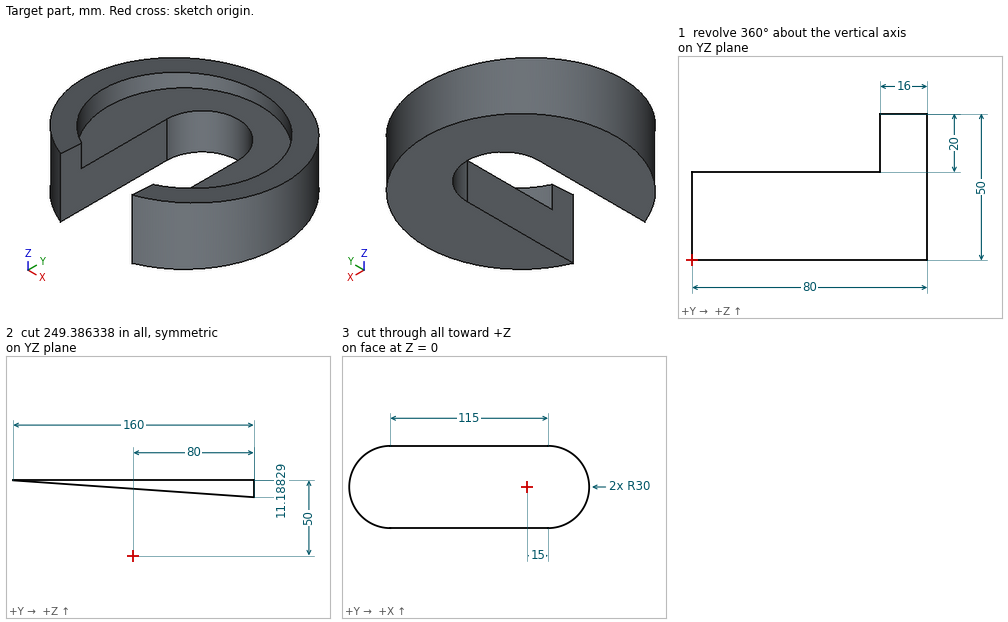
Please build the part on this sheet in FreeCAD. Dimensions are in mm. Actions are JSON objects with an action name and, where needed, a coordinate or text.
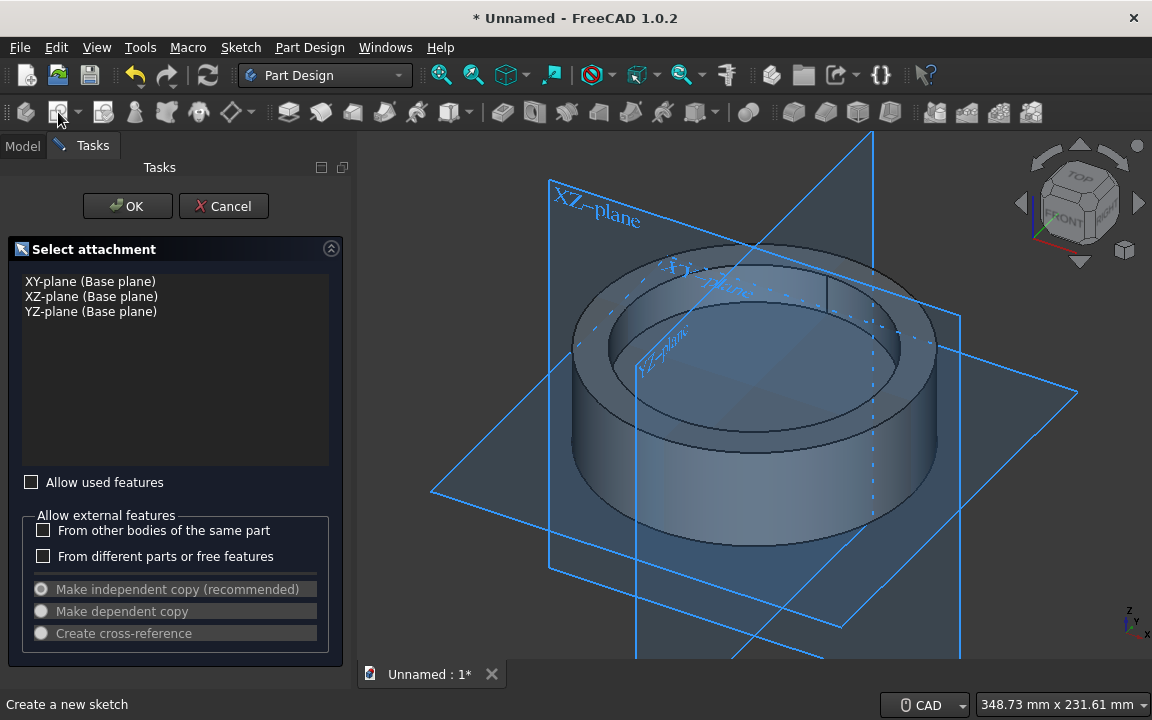
{"action": "left_click", "coordinate": [82, 312]}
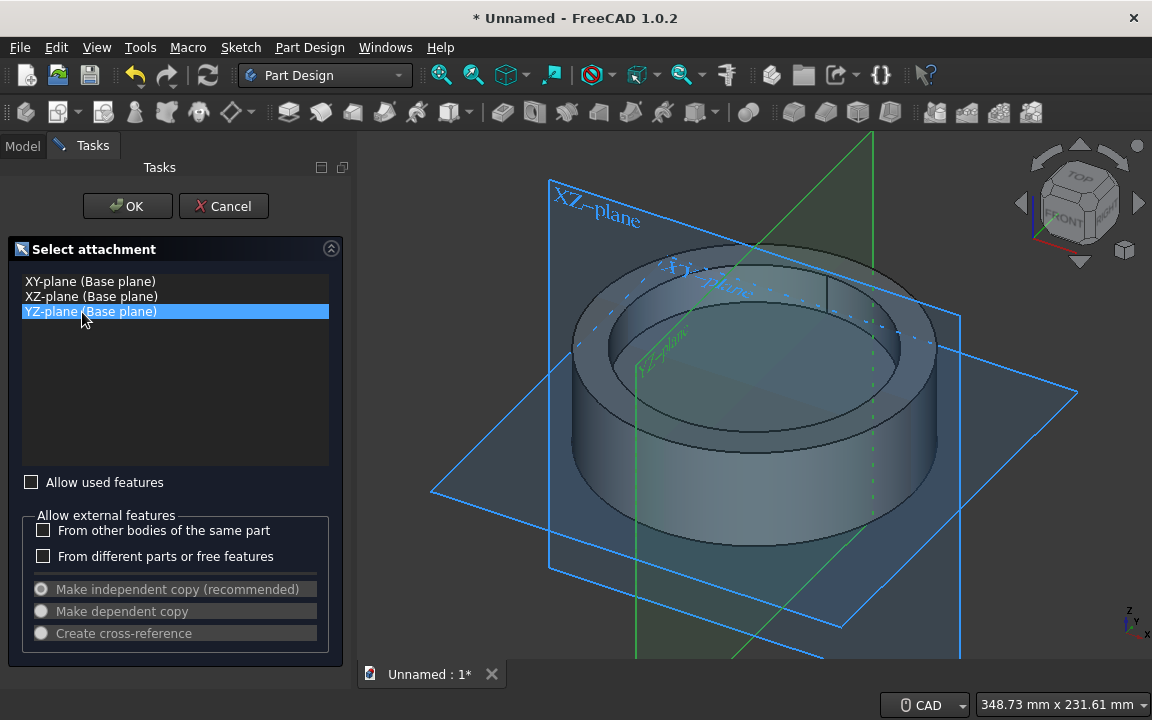
{"action": "left_click", "coordinate": [128, 206]}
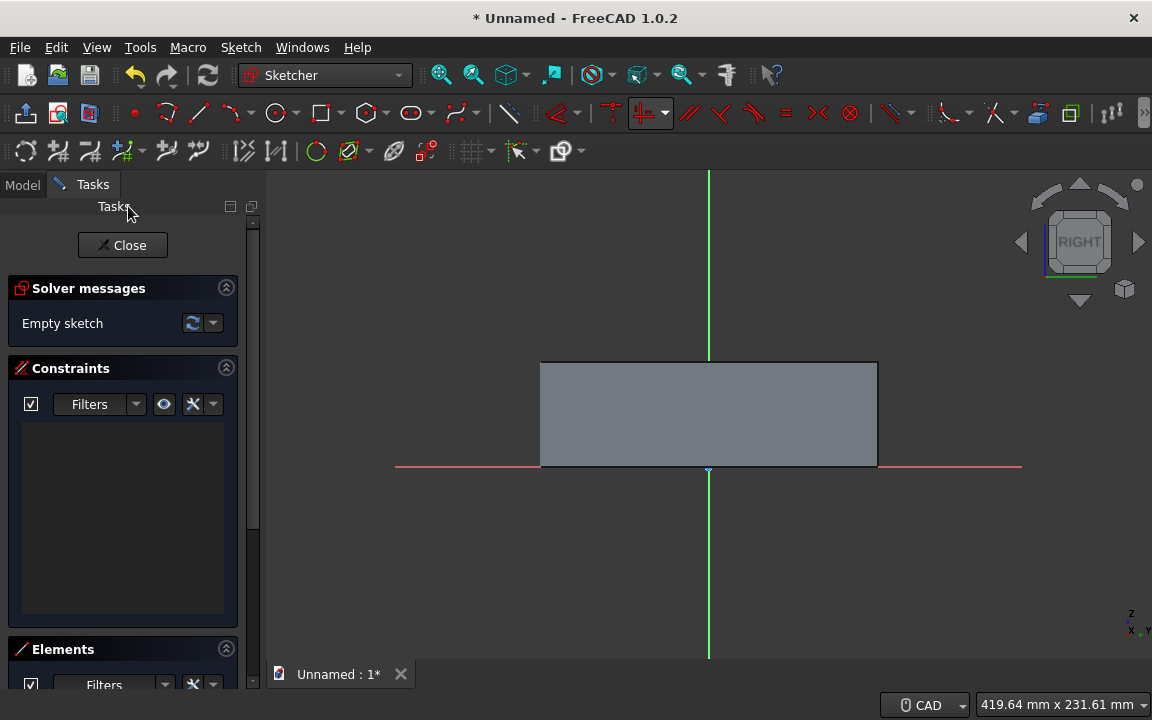
{"action": "left_click", "coordinate": [90, 114]}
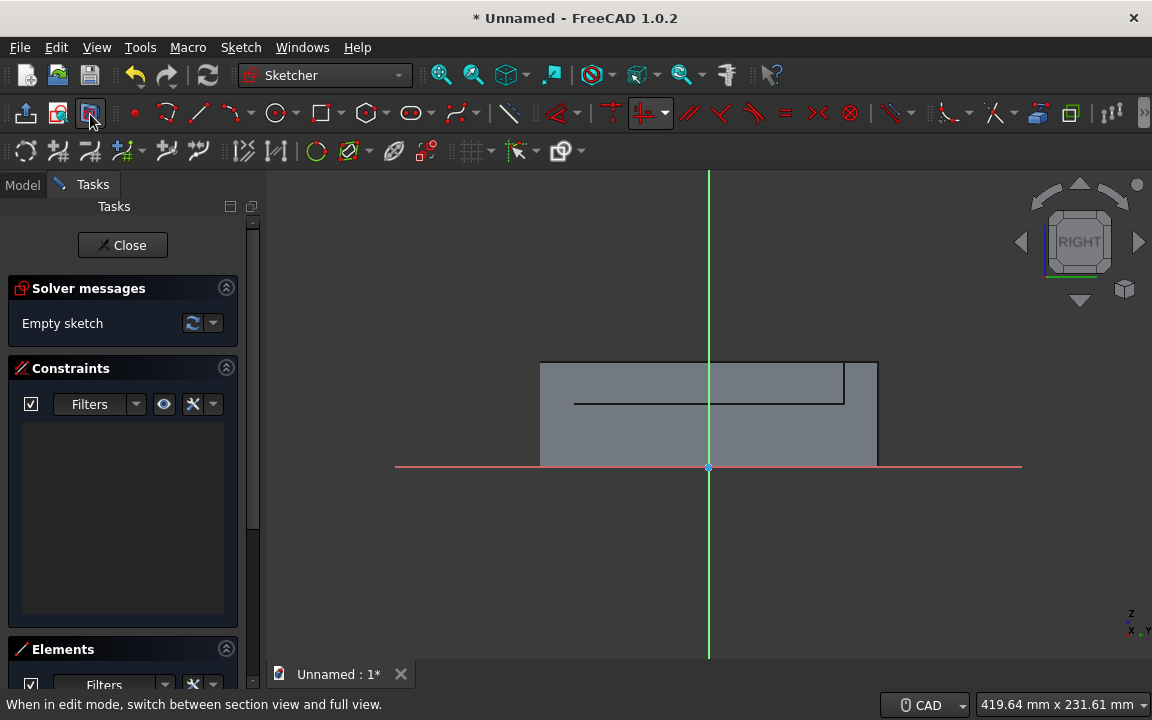
{"action": "scroll", "coordinate": [848, 414], "scroll_direction": "up", "scroll_amount": 2}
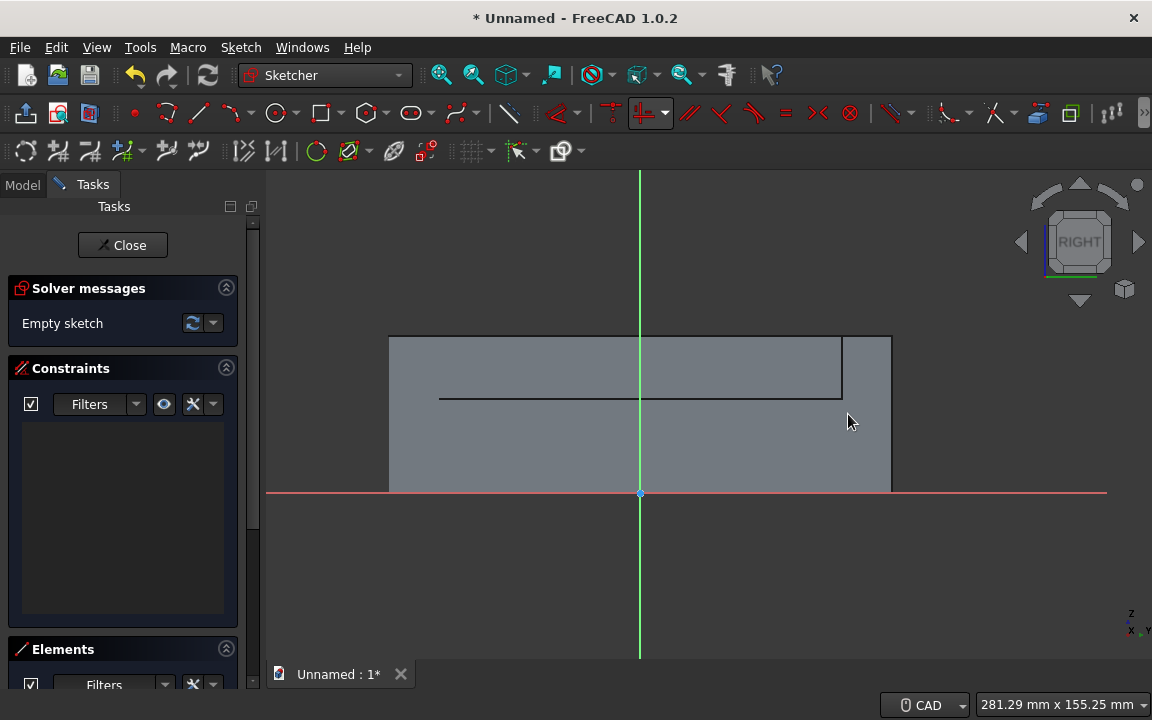
{"action": "left_click", "coordinate": [168, 114]}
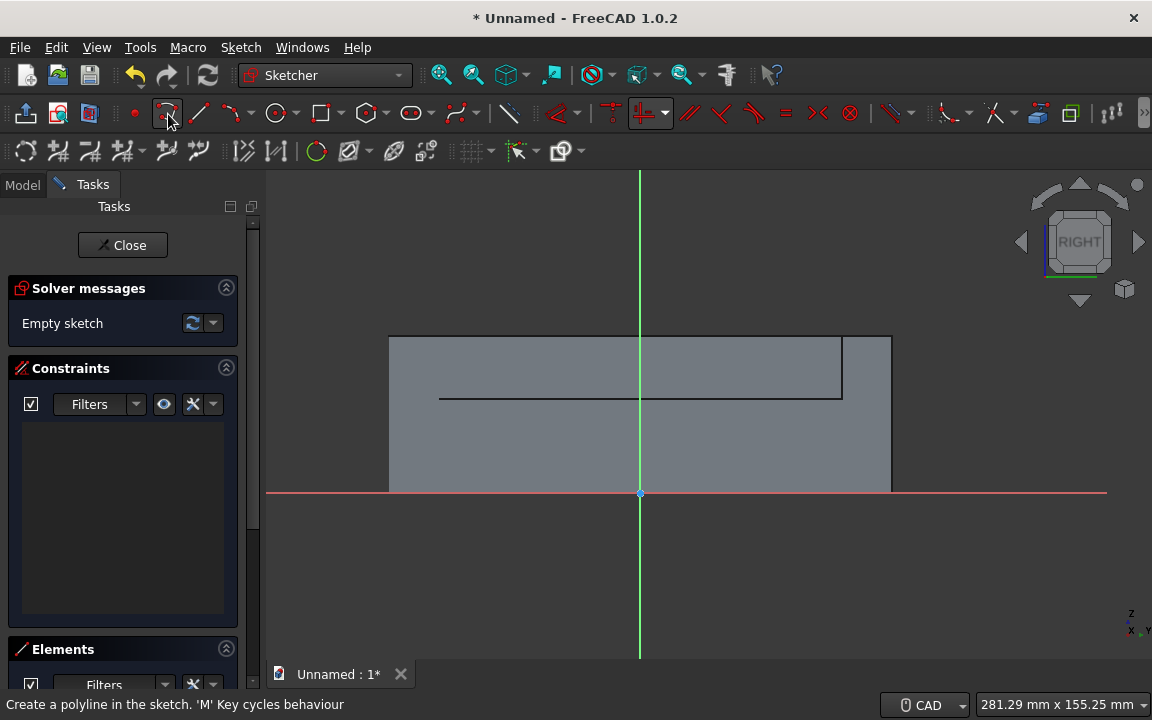
{"action": "left_click", "coordinate": [892, 371]}
{"action": "left_click", "coordinate": [892, 336]}
{"action": "left_click", "coordinate": [388, 336]}
{"action": "left_click", "coordinate": [892, 372]}
{"action": "key", "text": "Escape"}
{"action": "key", "text": "Escape"}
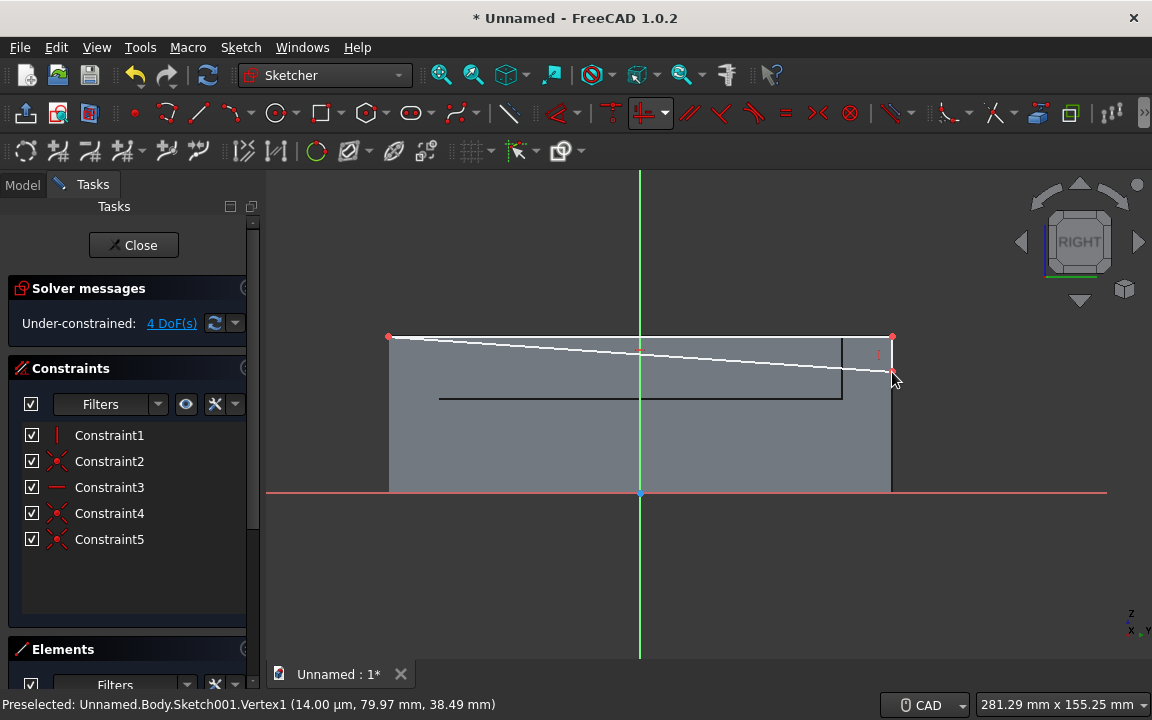
{"action": "left_click", "coordinate": [556, 114]}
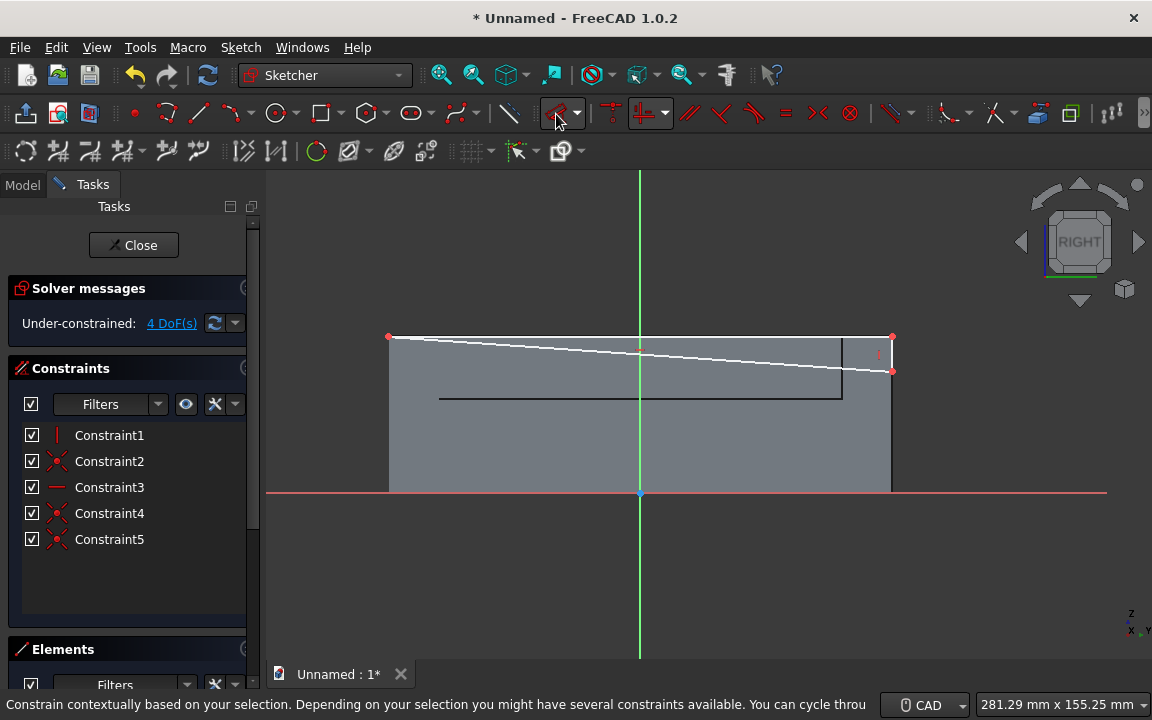
{"action": "left_click", "coordinate": [741, 337]}
{"action": "left_click", "coordinate": [524, 303]}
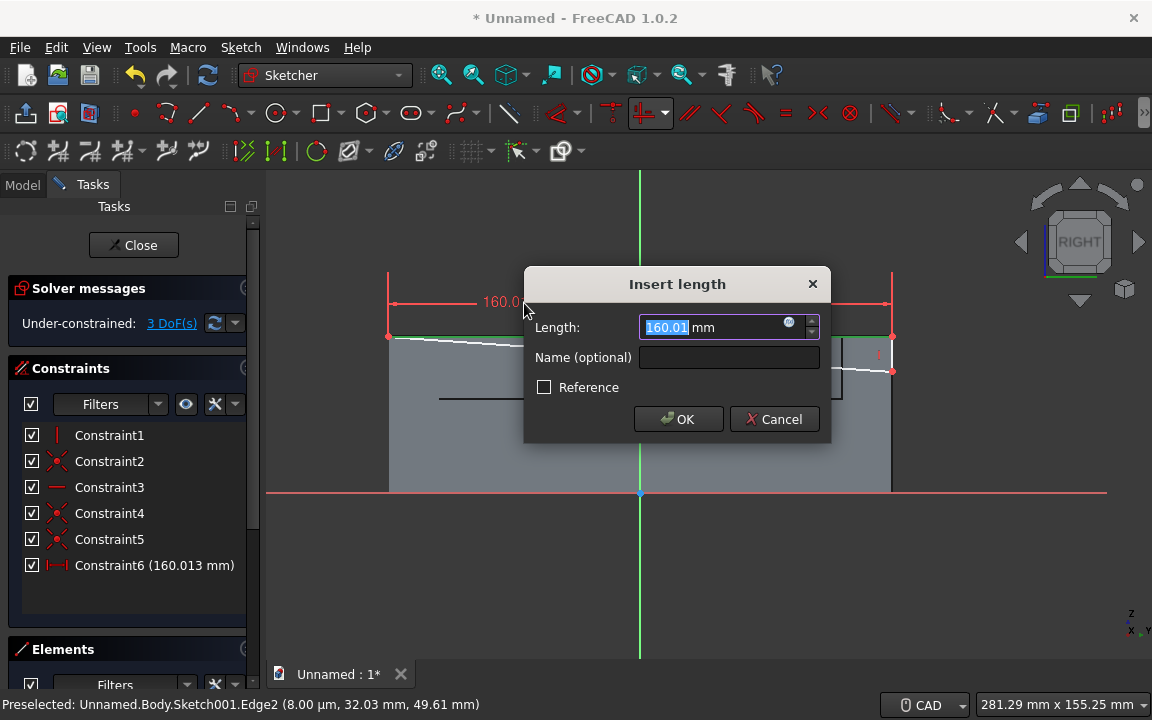
{"action": "type", "text": "160"}
{"action": "key", "text": "Return"}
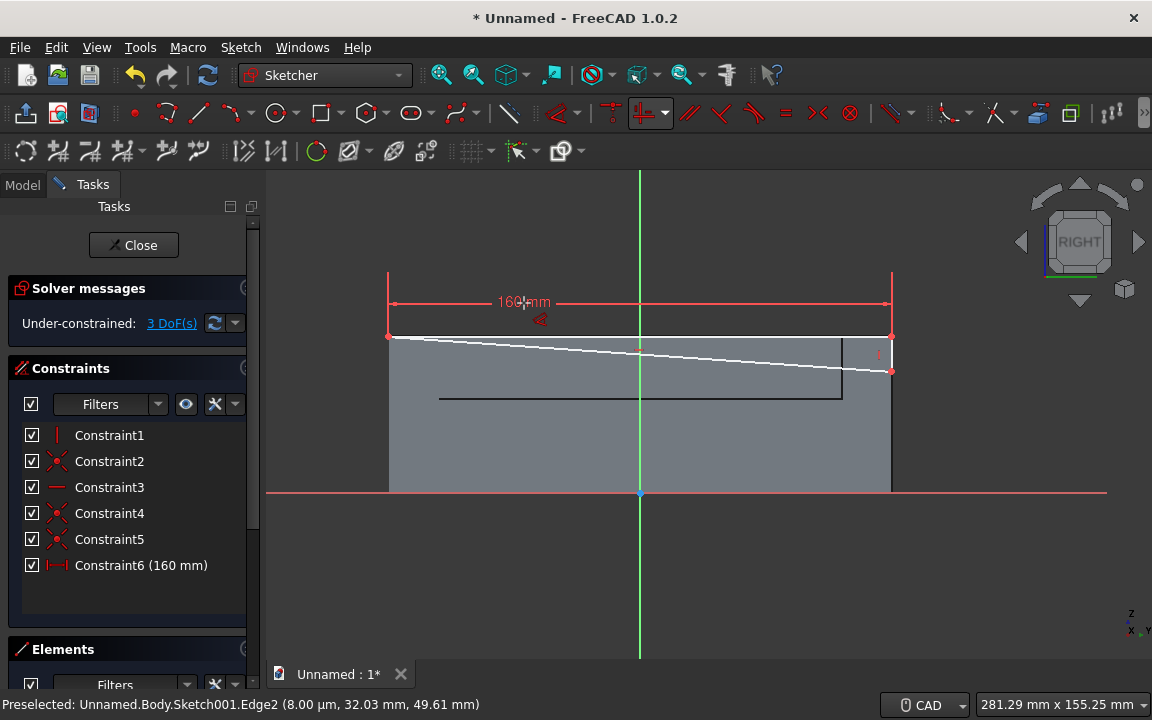
{"action": "left_click", "coordinate": [892, 372]}
{"action": "left_click", "coordinate": [766, 527]}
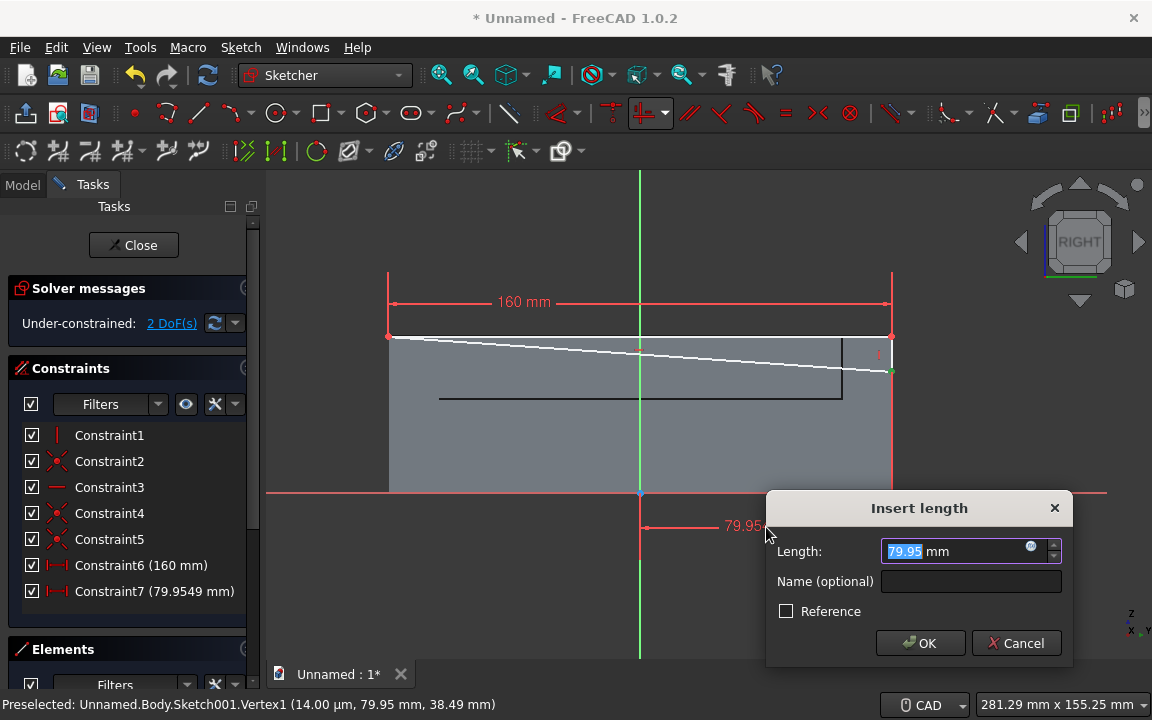
{"action": "type", "text": "80"}
{"action": "key", "text": "Return"}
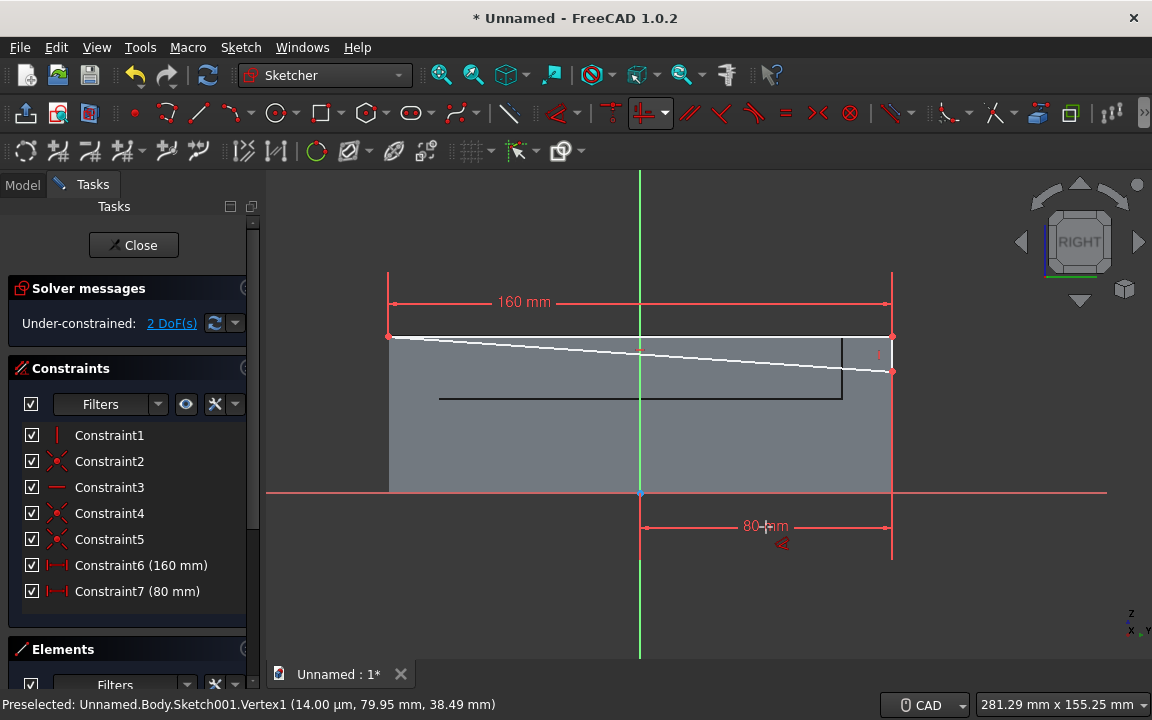
{"action": "left_click", "coordinate": [892, 337]}
{"action": "left_click", "coordinate": [926, 415]}